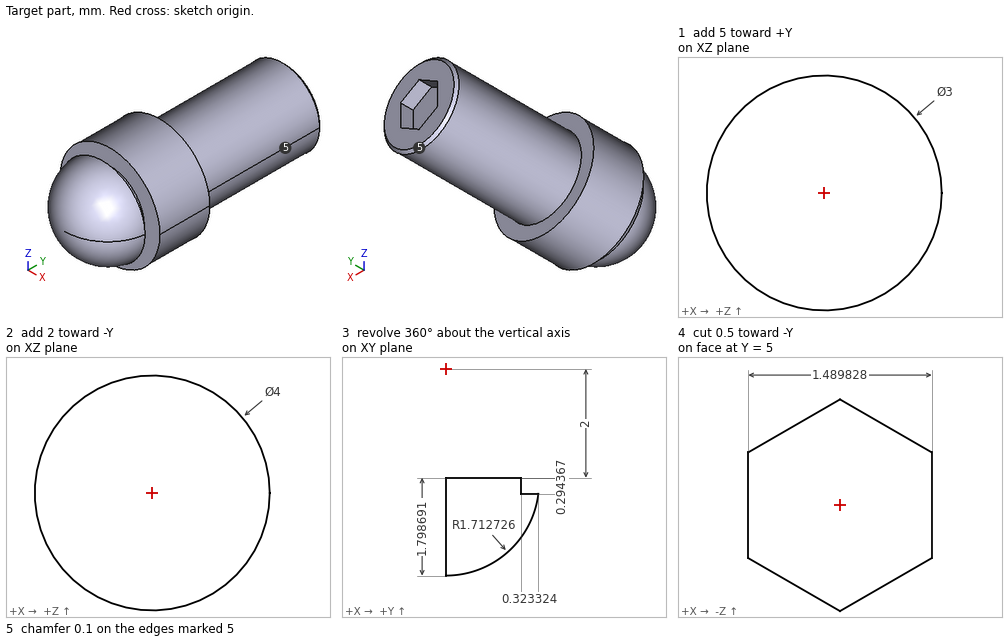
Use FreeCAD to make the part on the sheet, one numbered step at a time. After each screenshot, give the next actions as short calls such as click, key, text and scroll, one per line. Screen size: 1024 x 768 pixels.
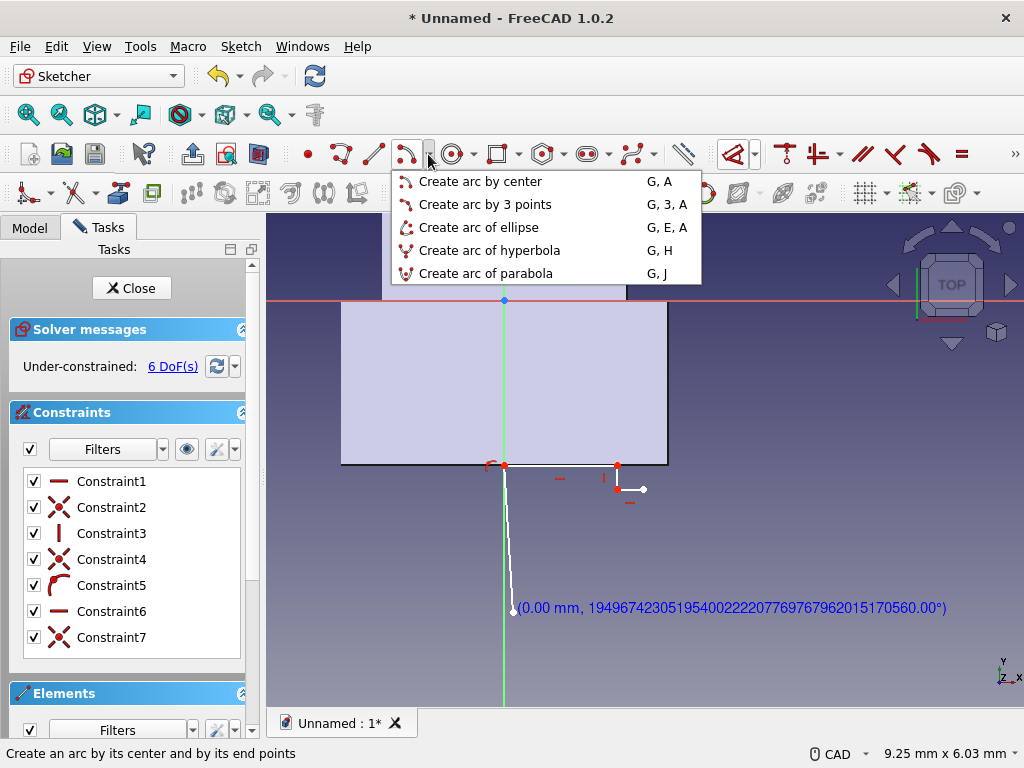
click(546, 204)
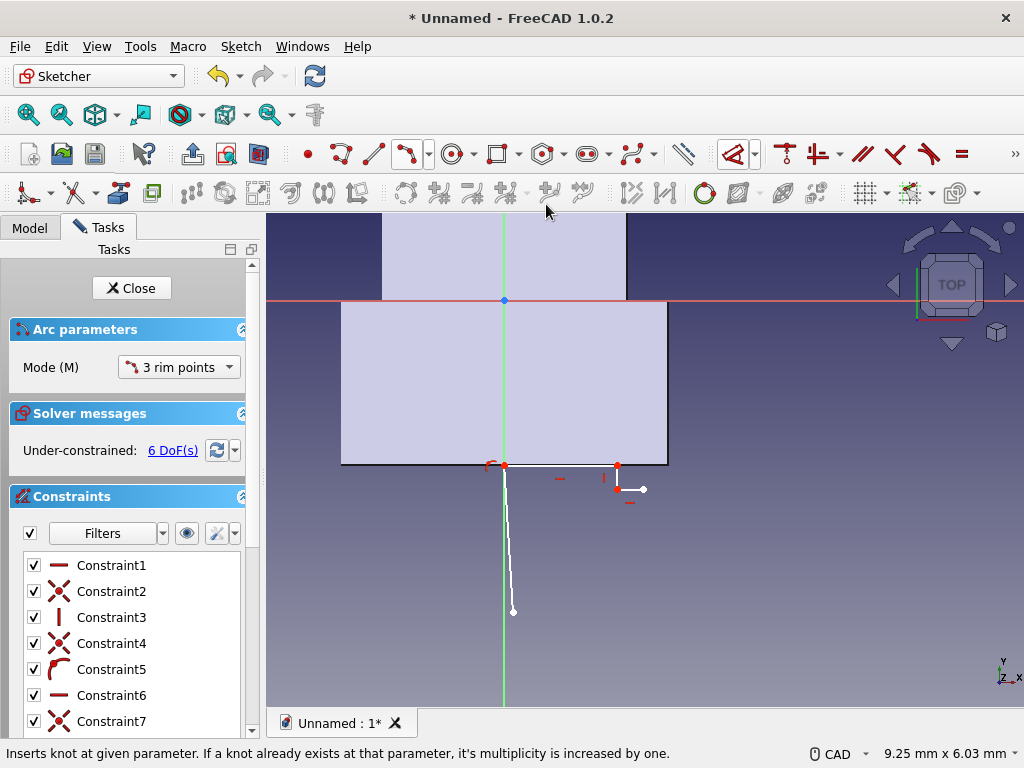
click(513, 613)
click(643, 490)
click(597, 577)
key(Escape)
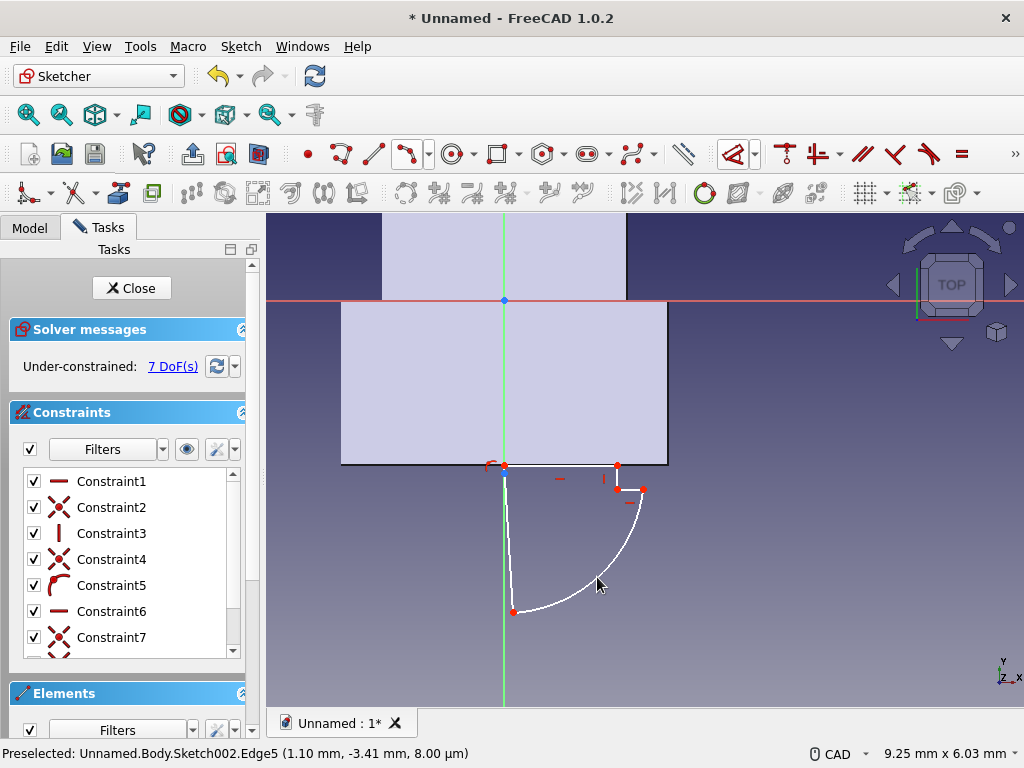
click(507, 510)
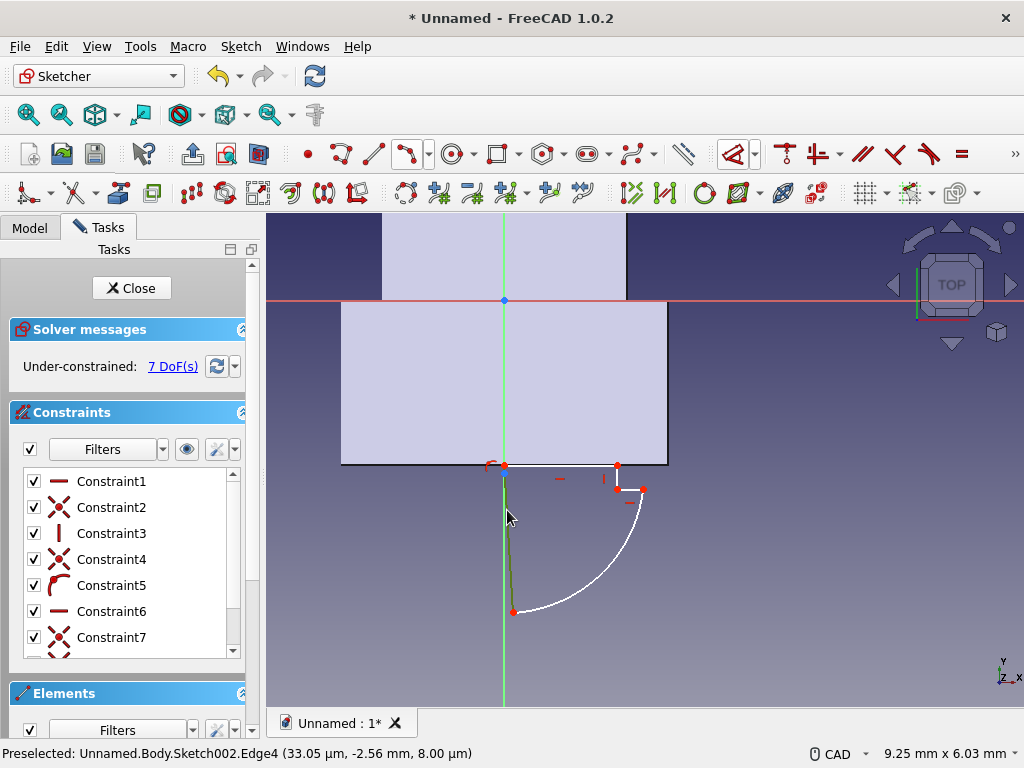
key(v)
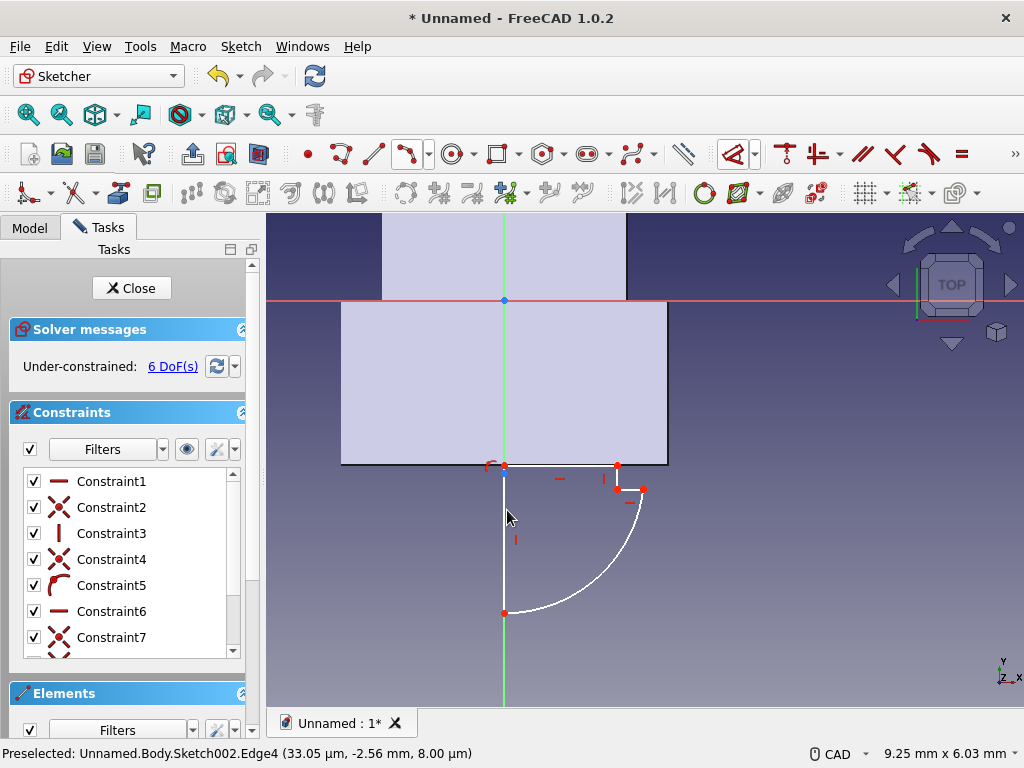
scroll(504, 473, up, 3)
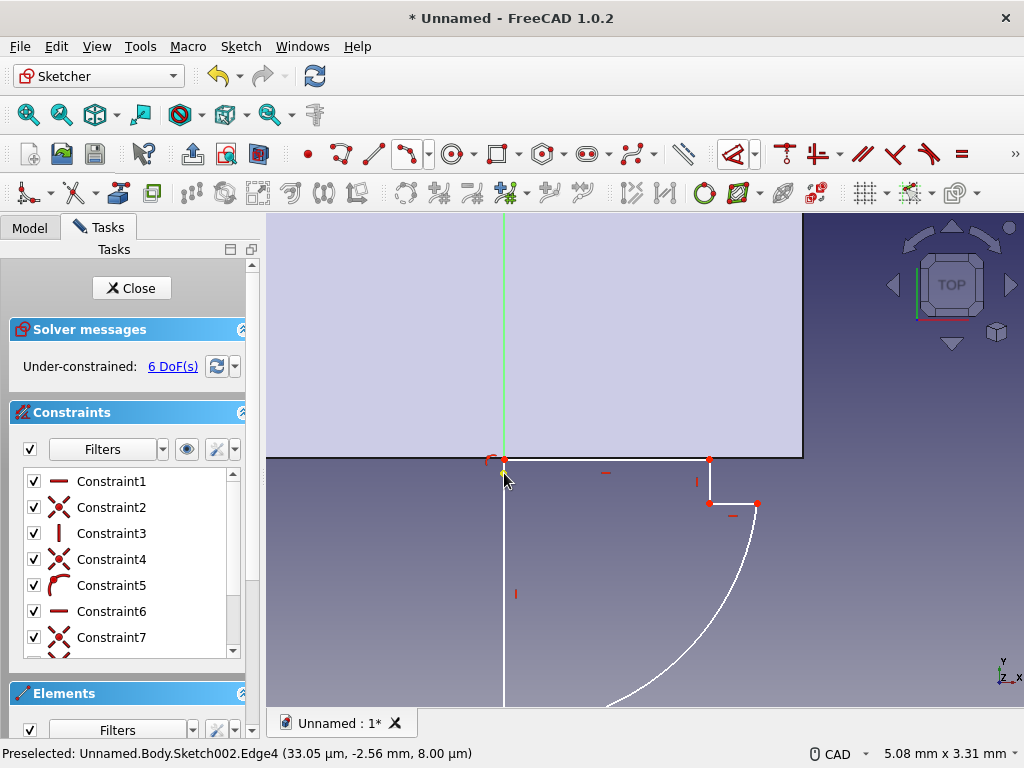
click(504, 473)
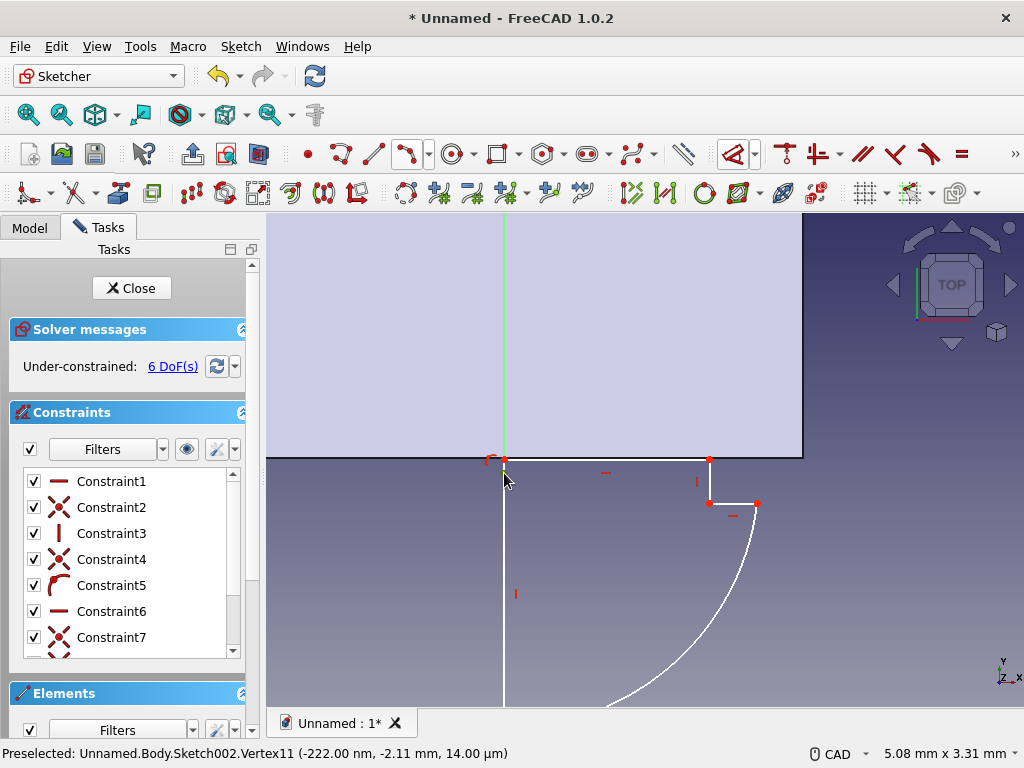
click(504, 429)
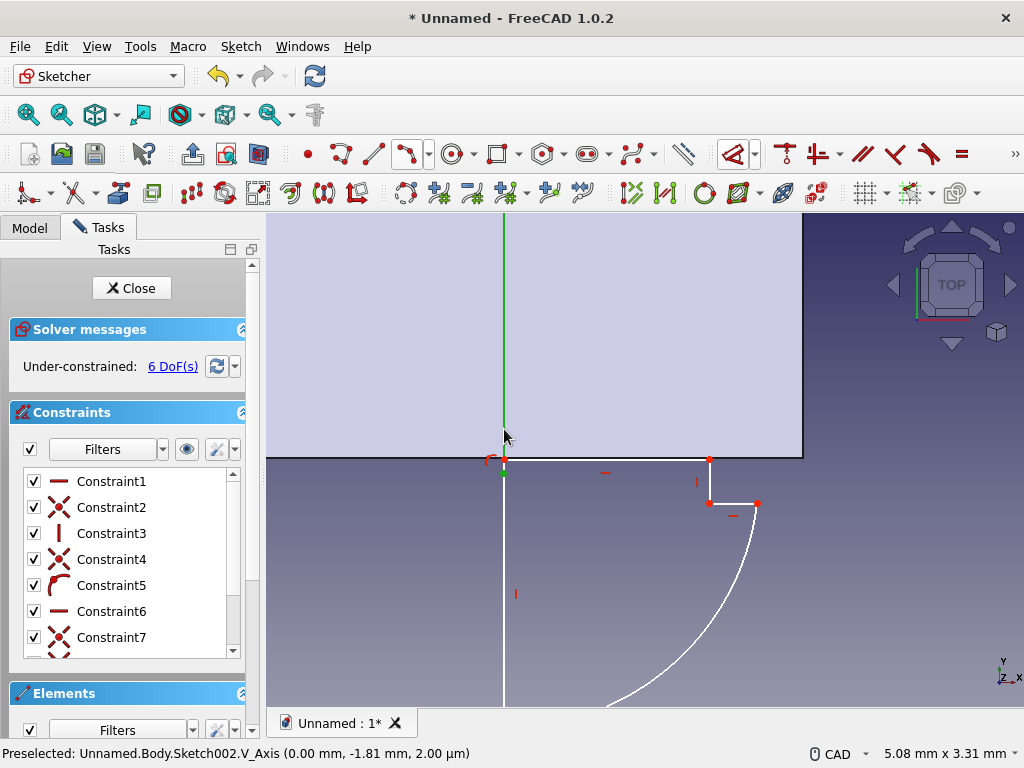
key(c)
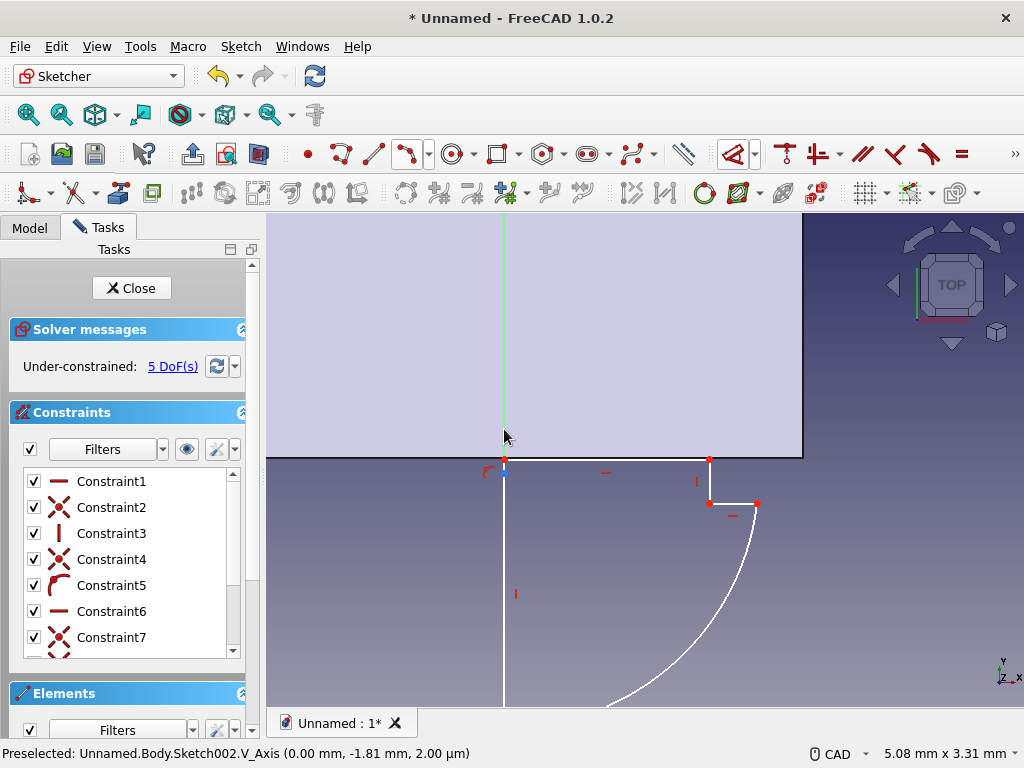
click(721, 607)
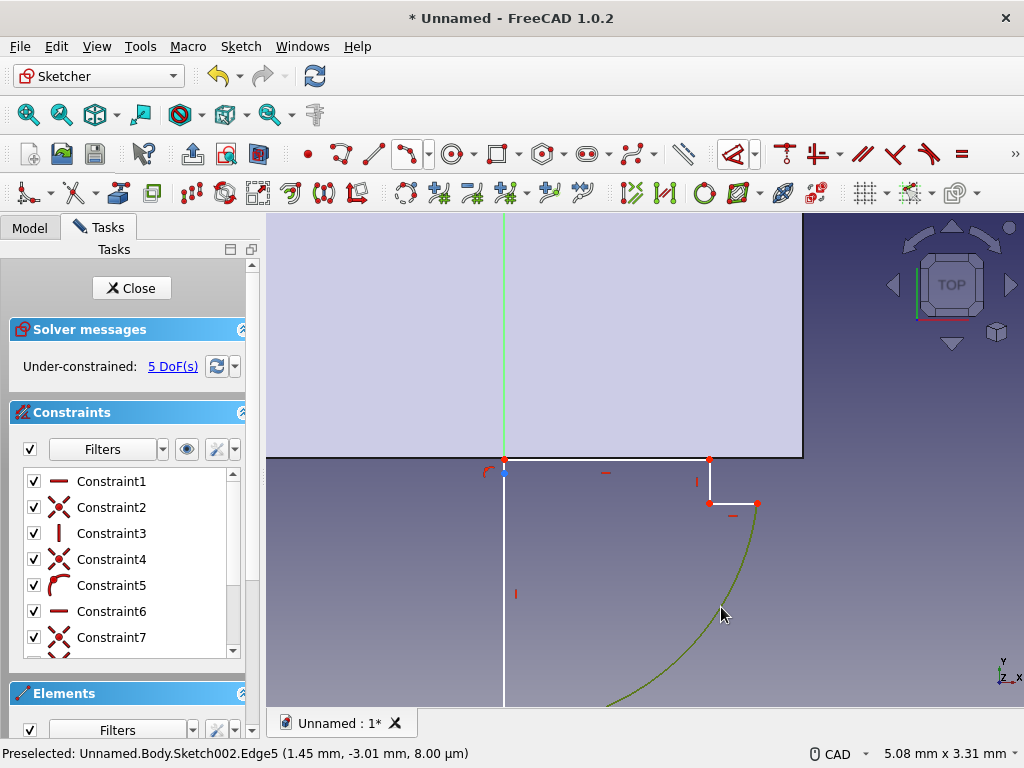
click(754, 154)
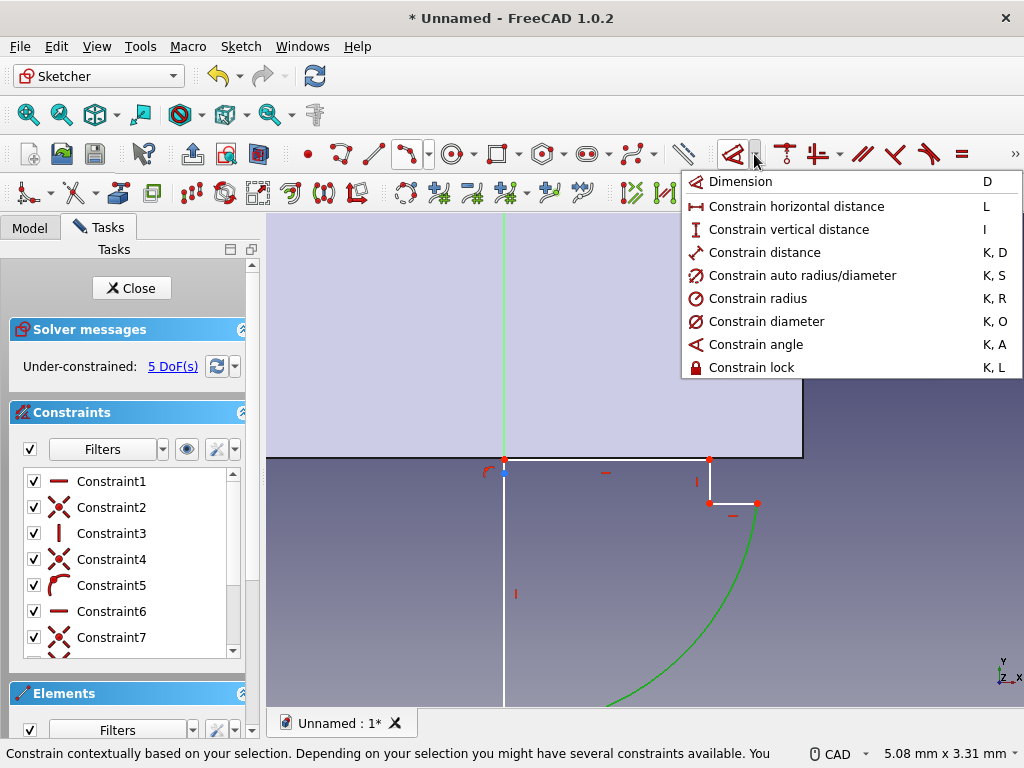
click(852, 298)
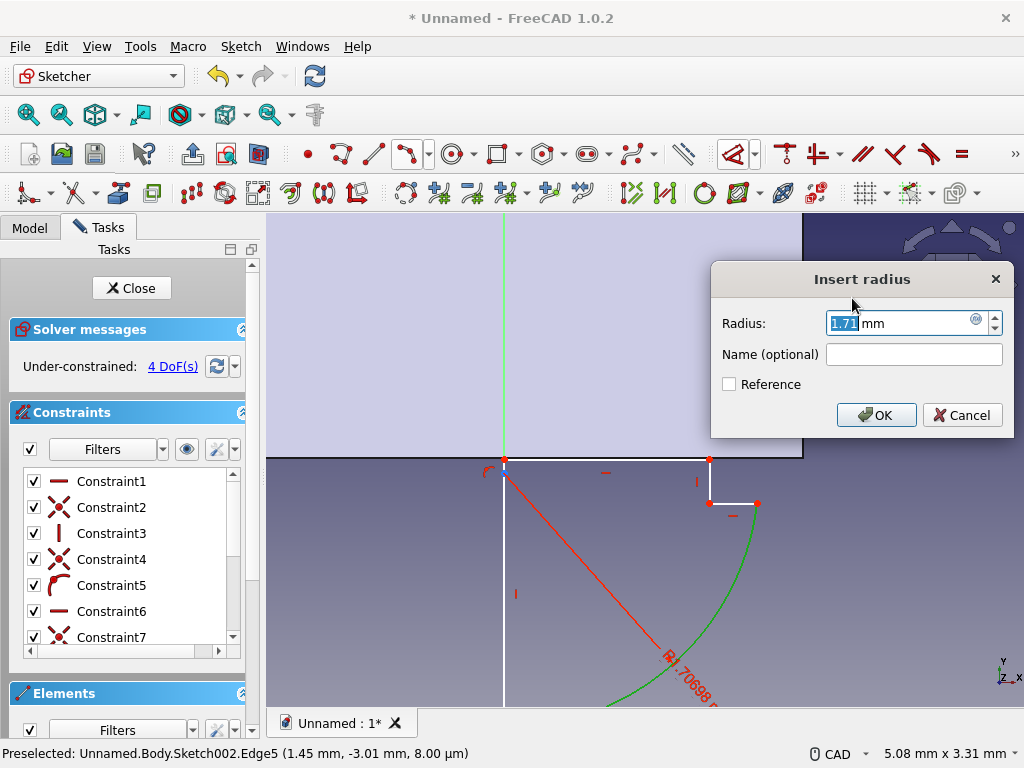
text(1.712726)
key(Return)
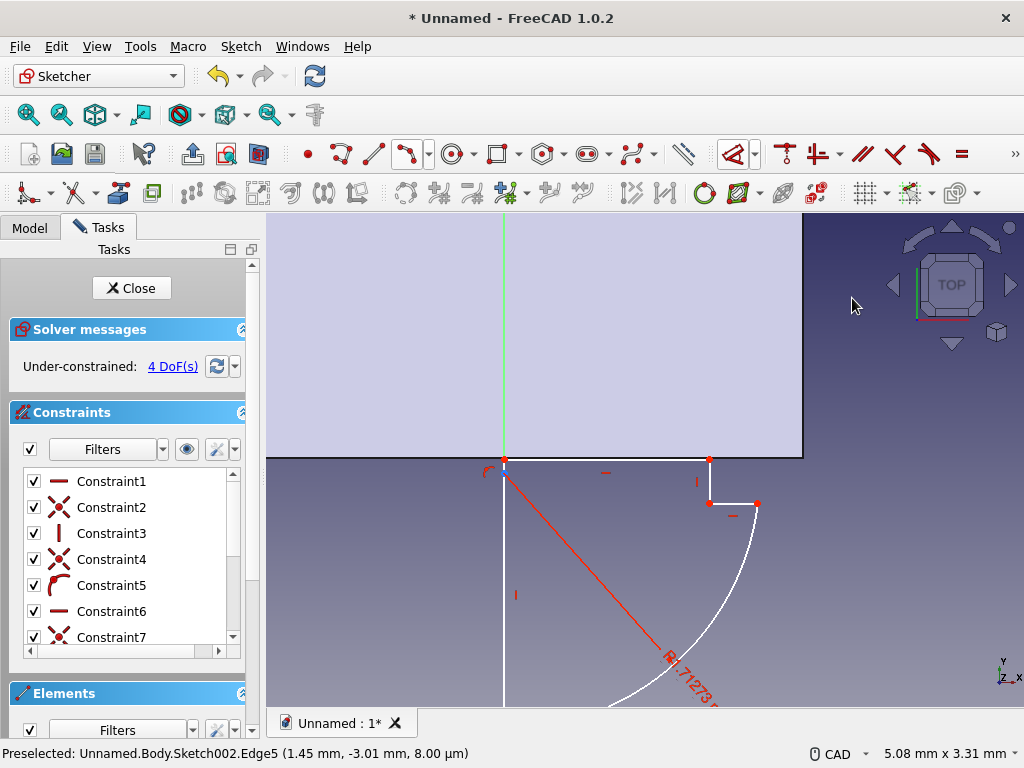
click(710, 460)